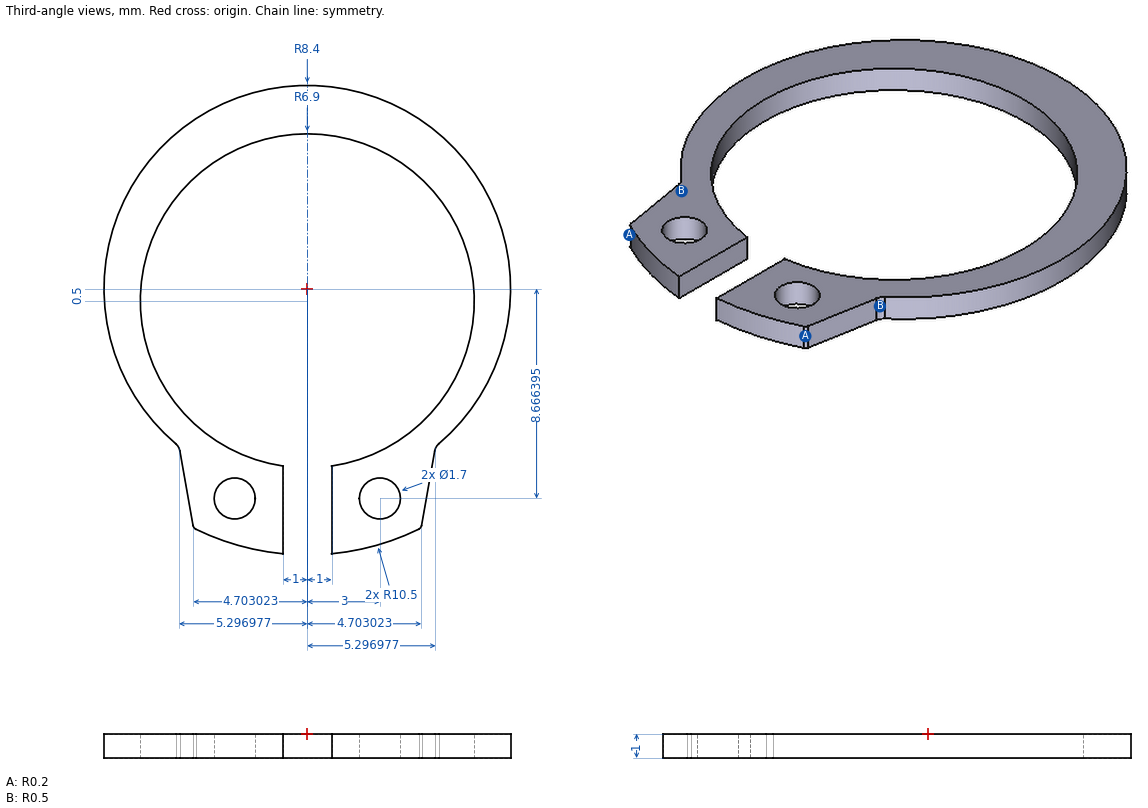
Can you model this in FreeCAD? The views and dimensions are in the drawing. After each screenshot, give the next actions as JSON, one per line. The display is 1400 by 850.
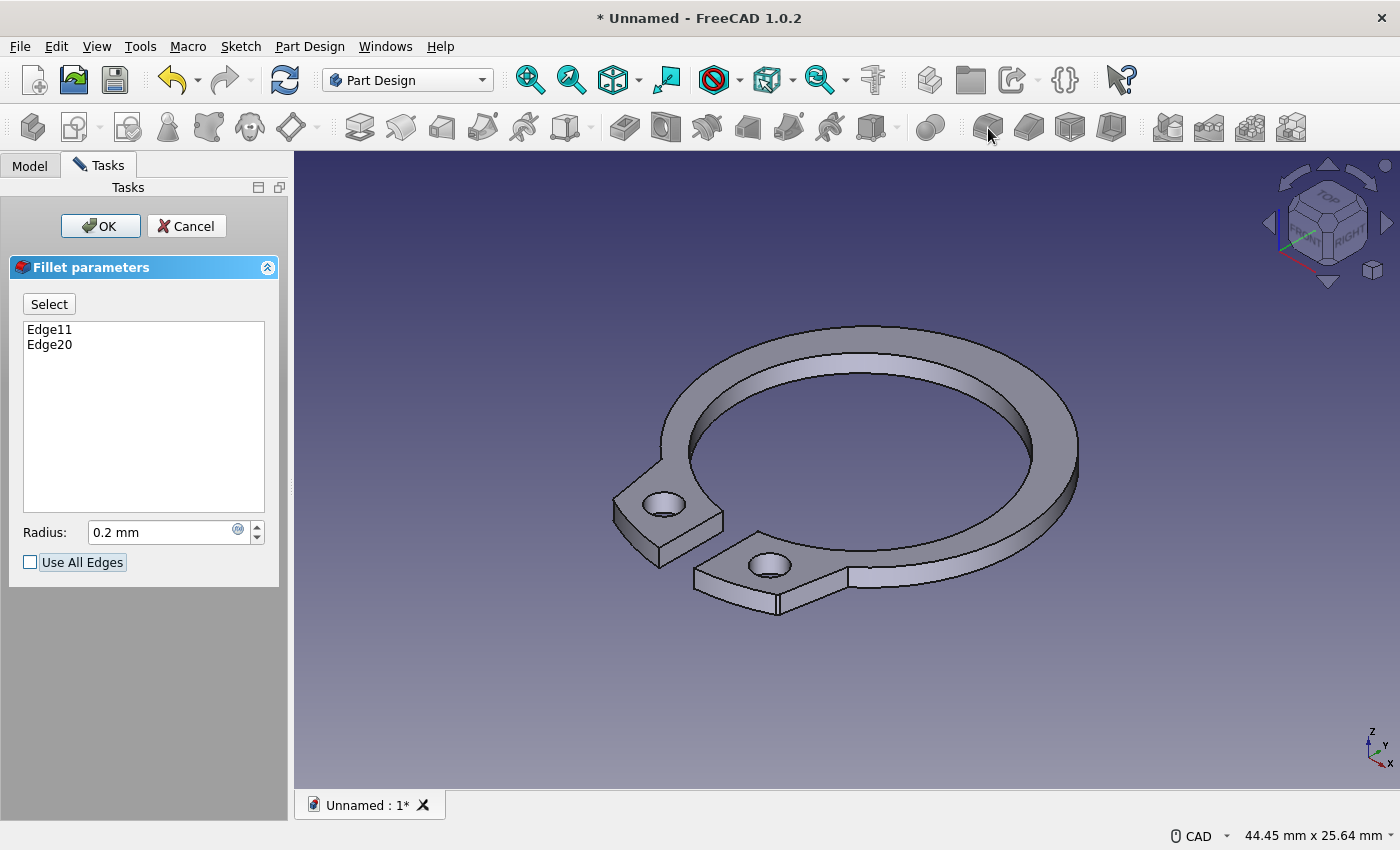
{"action": "left_click", "coordinate": [101, 226]}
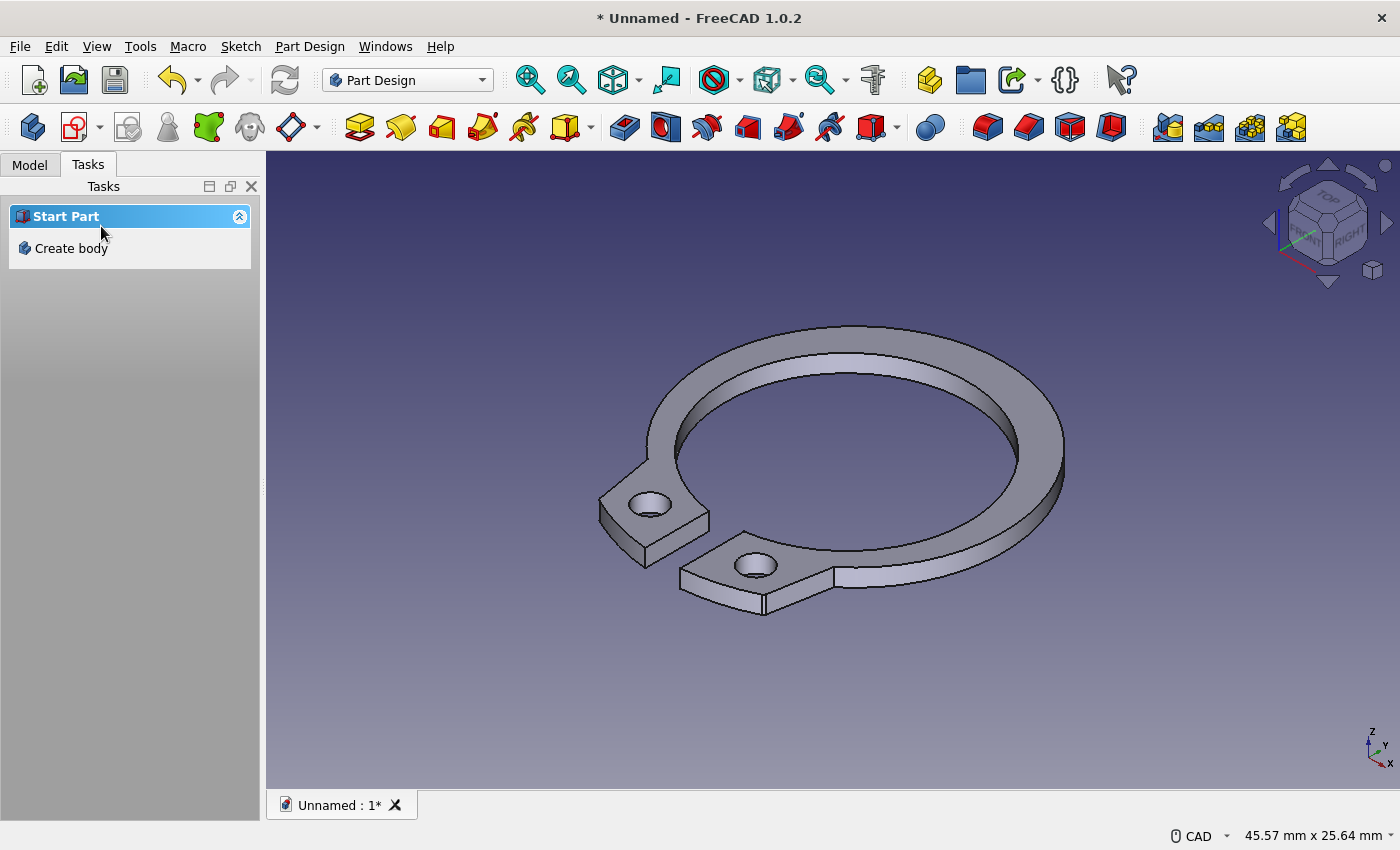
{"action": "key", "text": "2"}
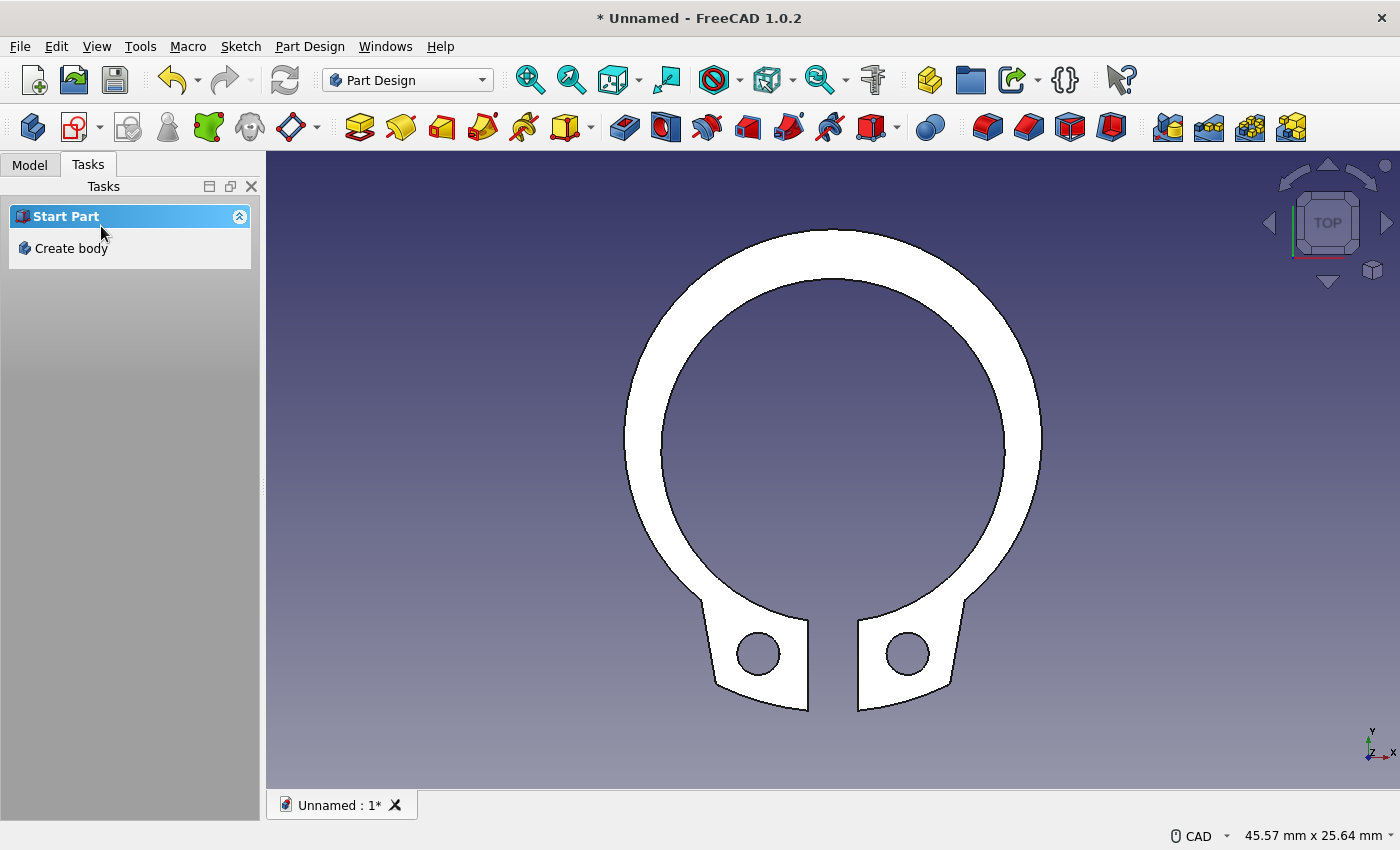
{"action": "key", "text": "0"}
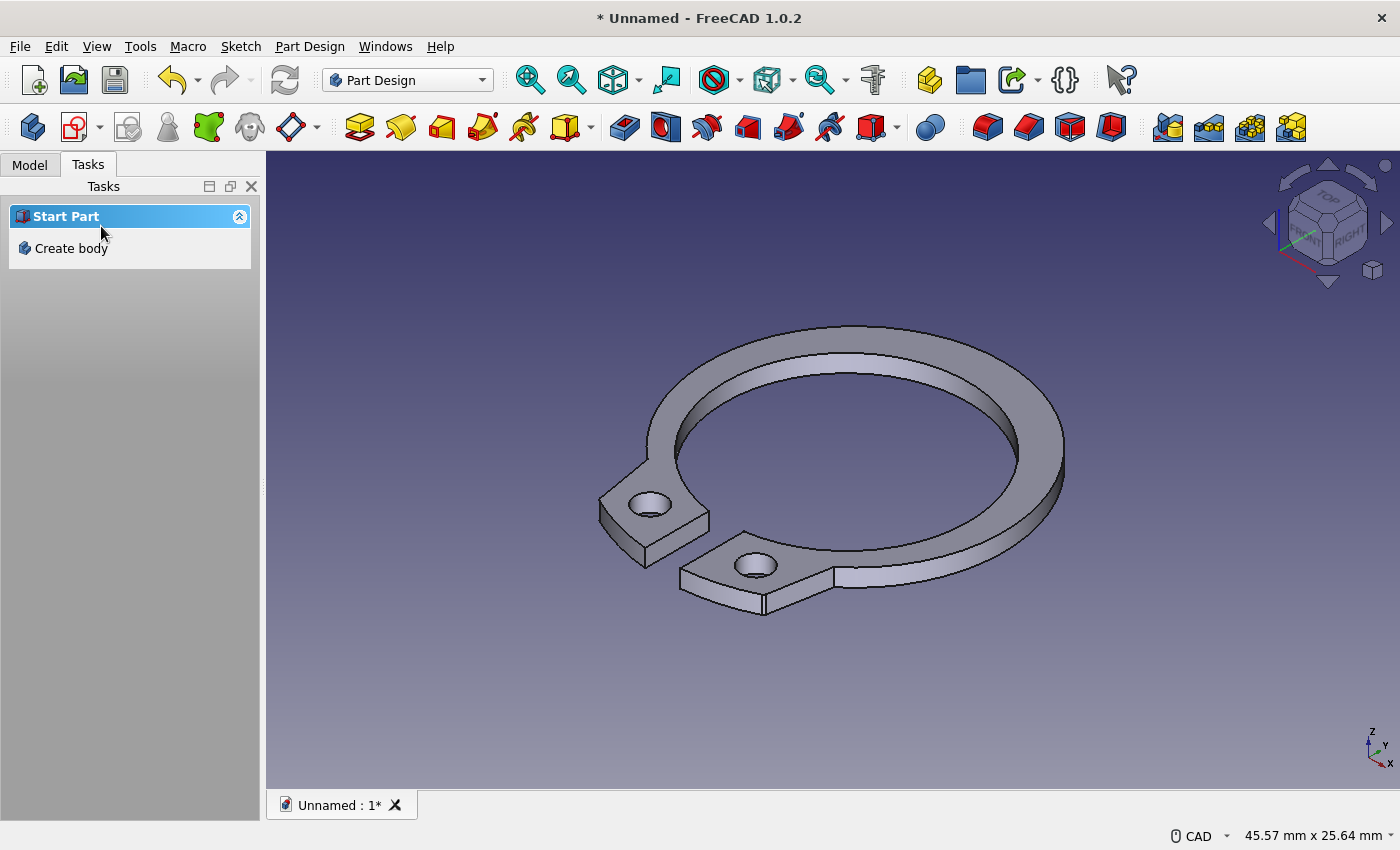
{"action": "key", "text": "1"}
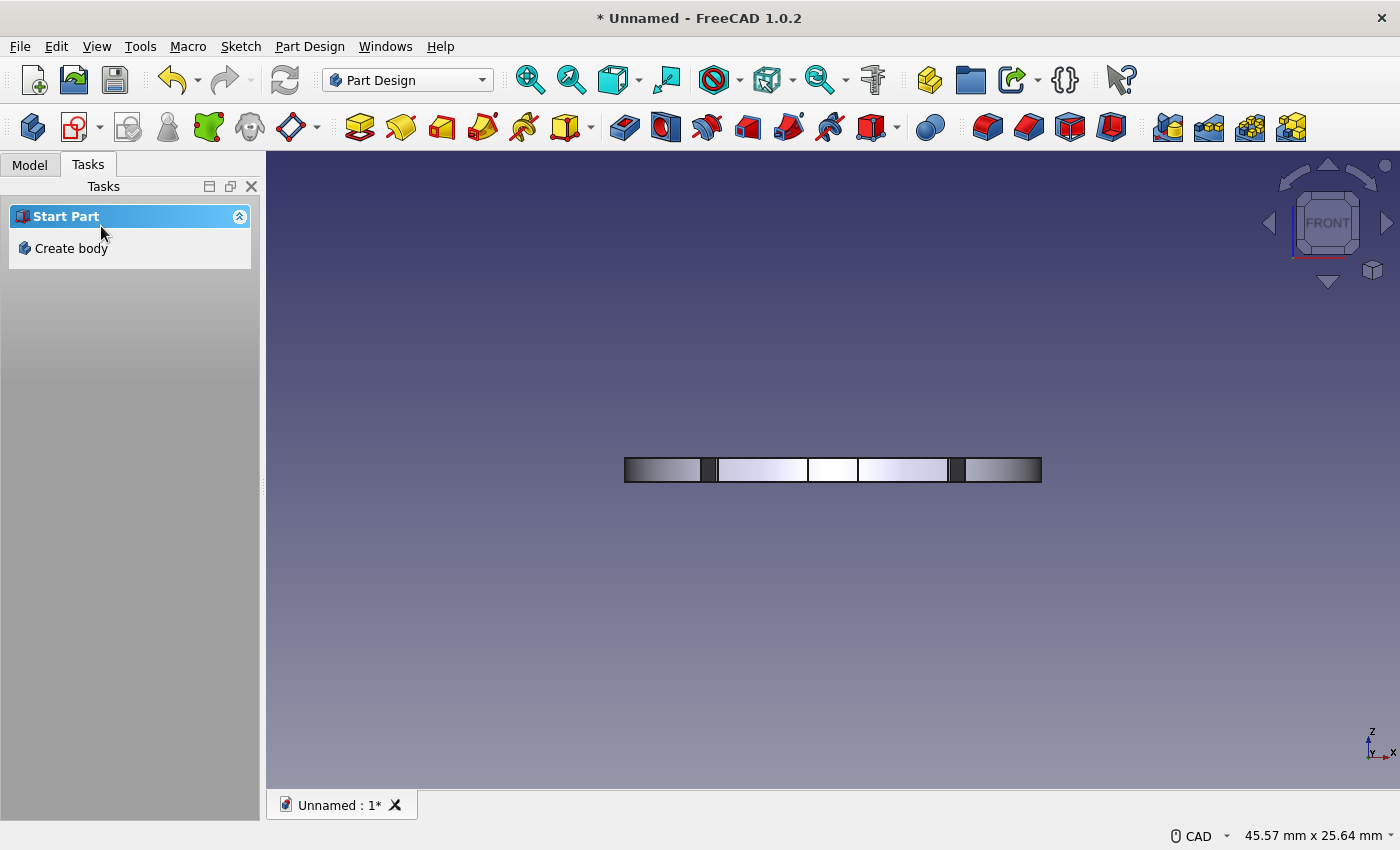
{"action": "left_click", "coordinate": [531, 80]}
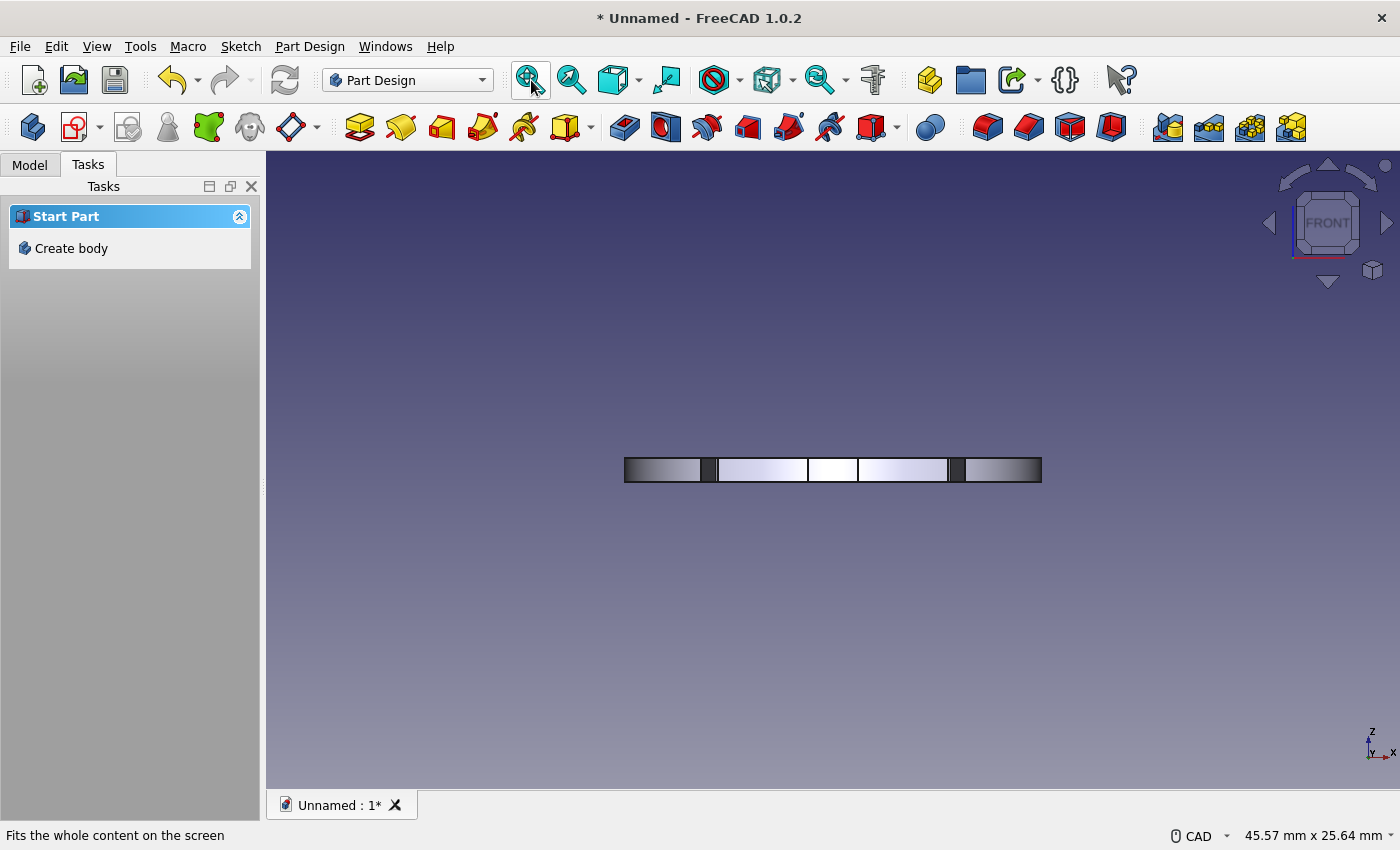
{"action": "key", "text": "3"}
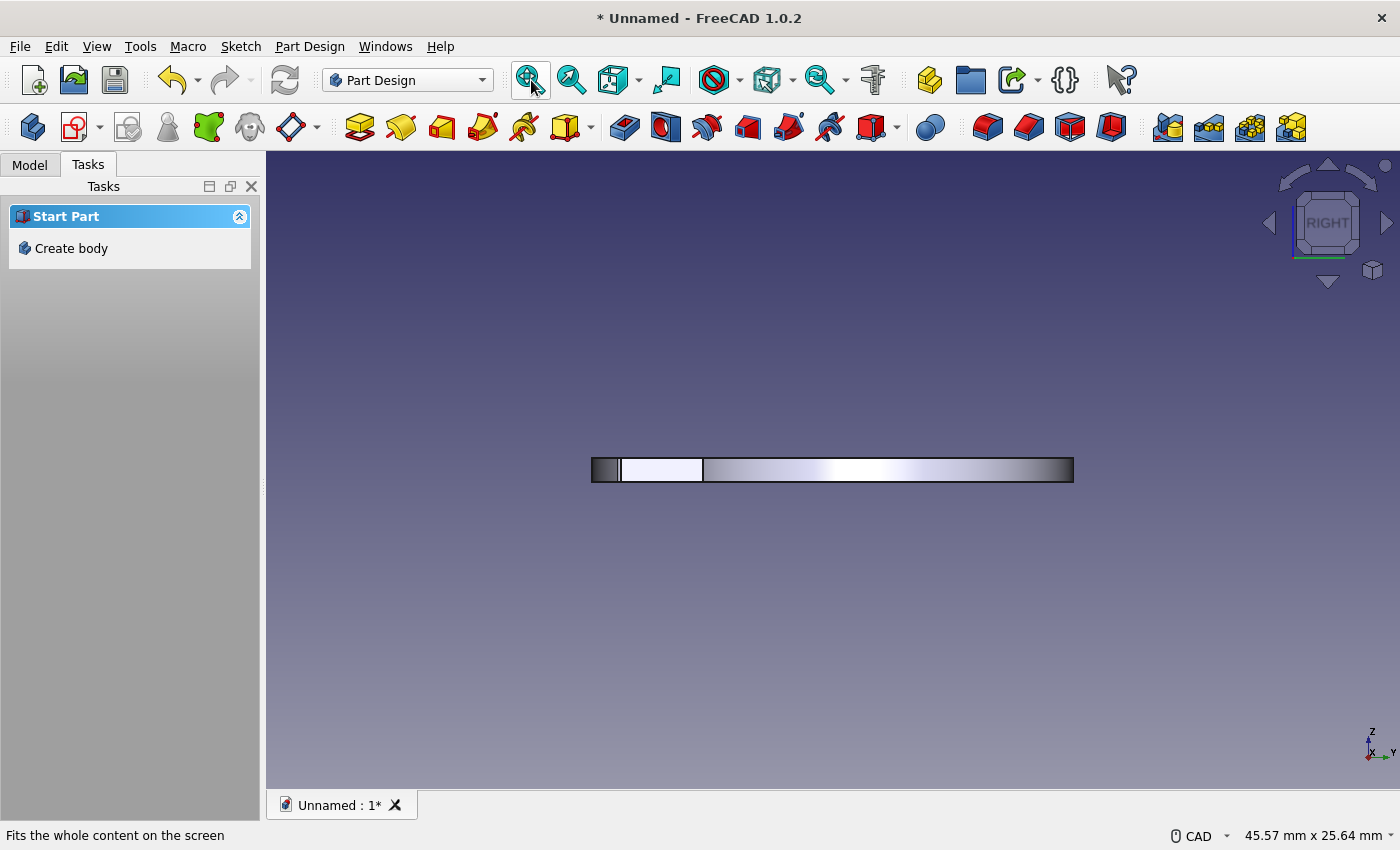
{"action": "left_click", "coordinate": [531, 80]}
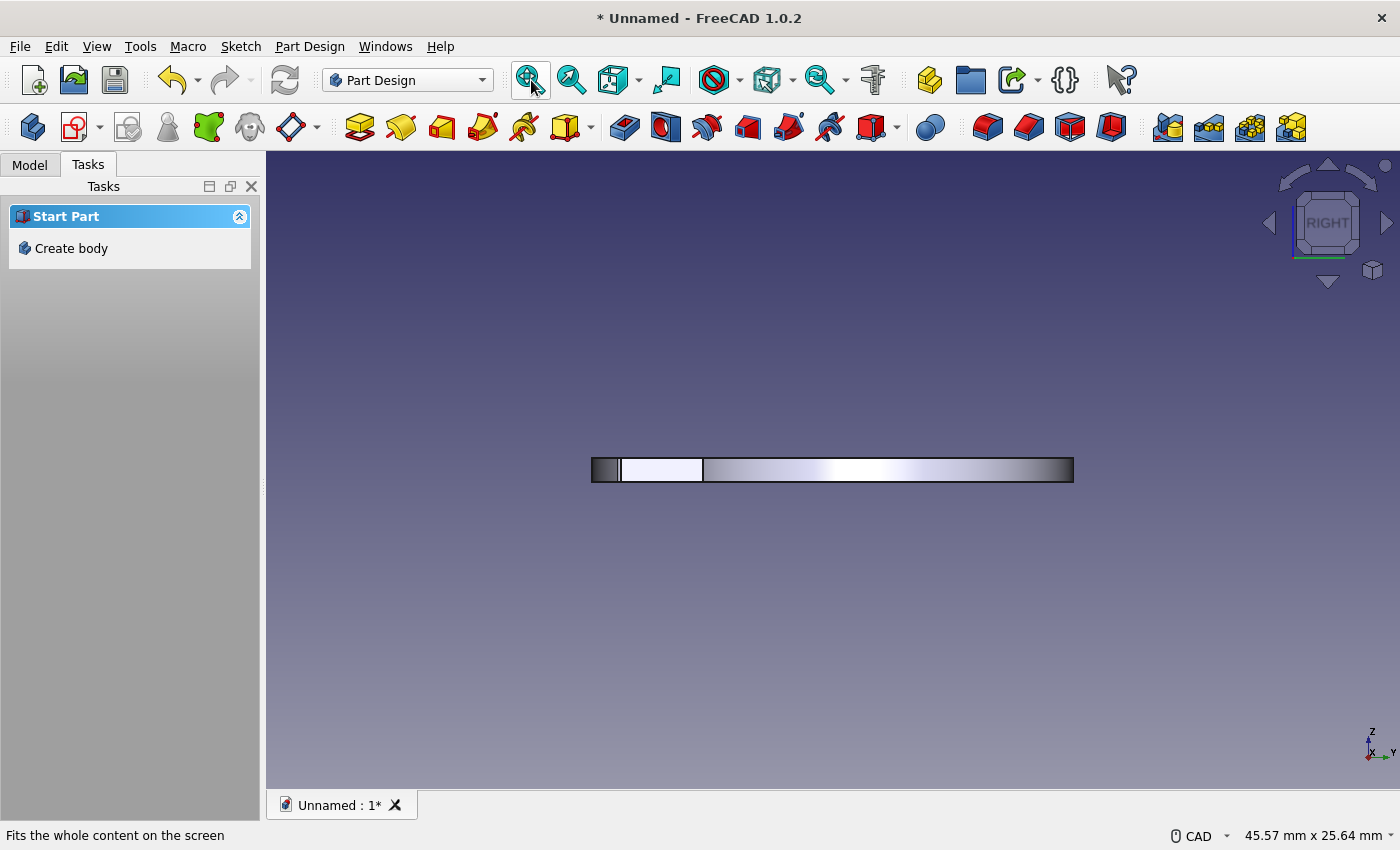
{"action": "key", "text": "5"}